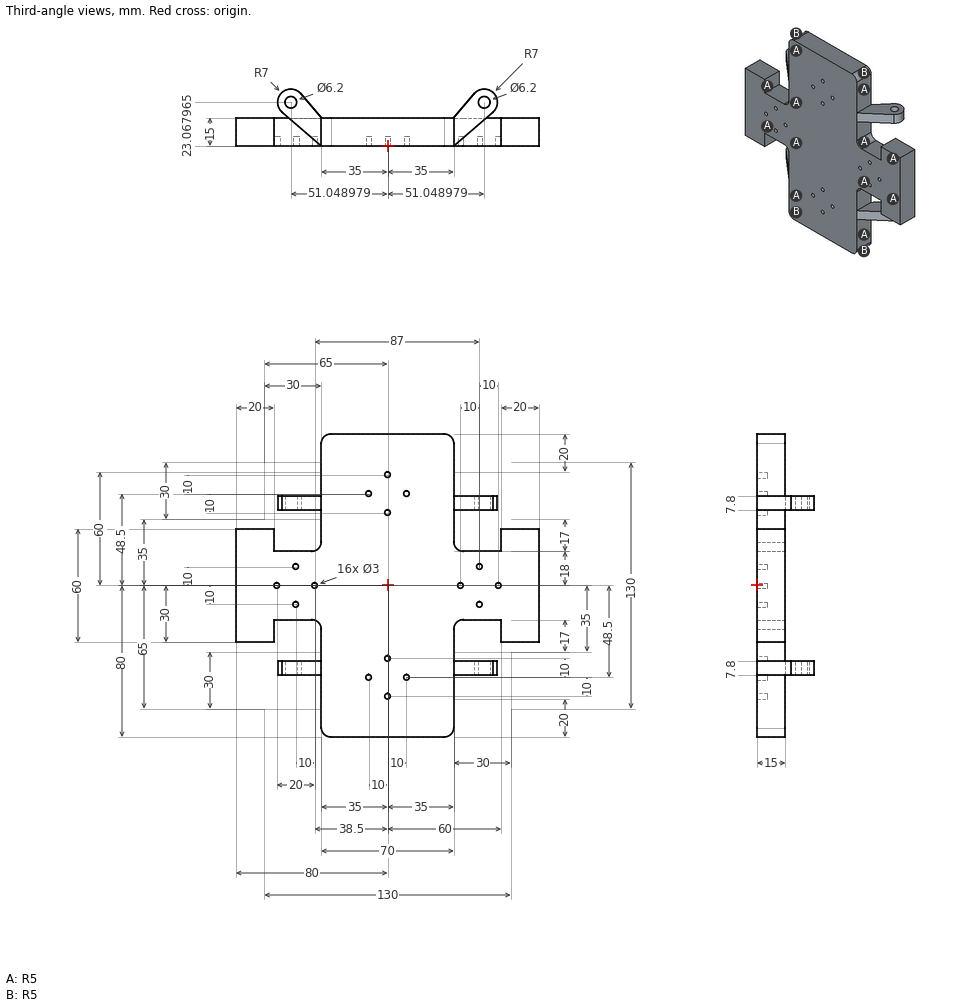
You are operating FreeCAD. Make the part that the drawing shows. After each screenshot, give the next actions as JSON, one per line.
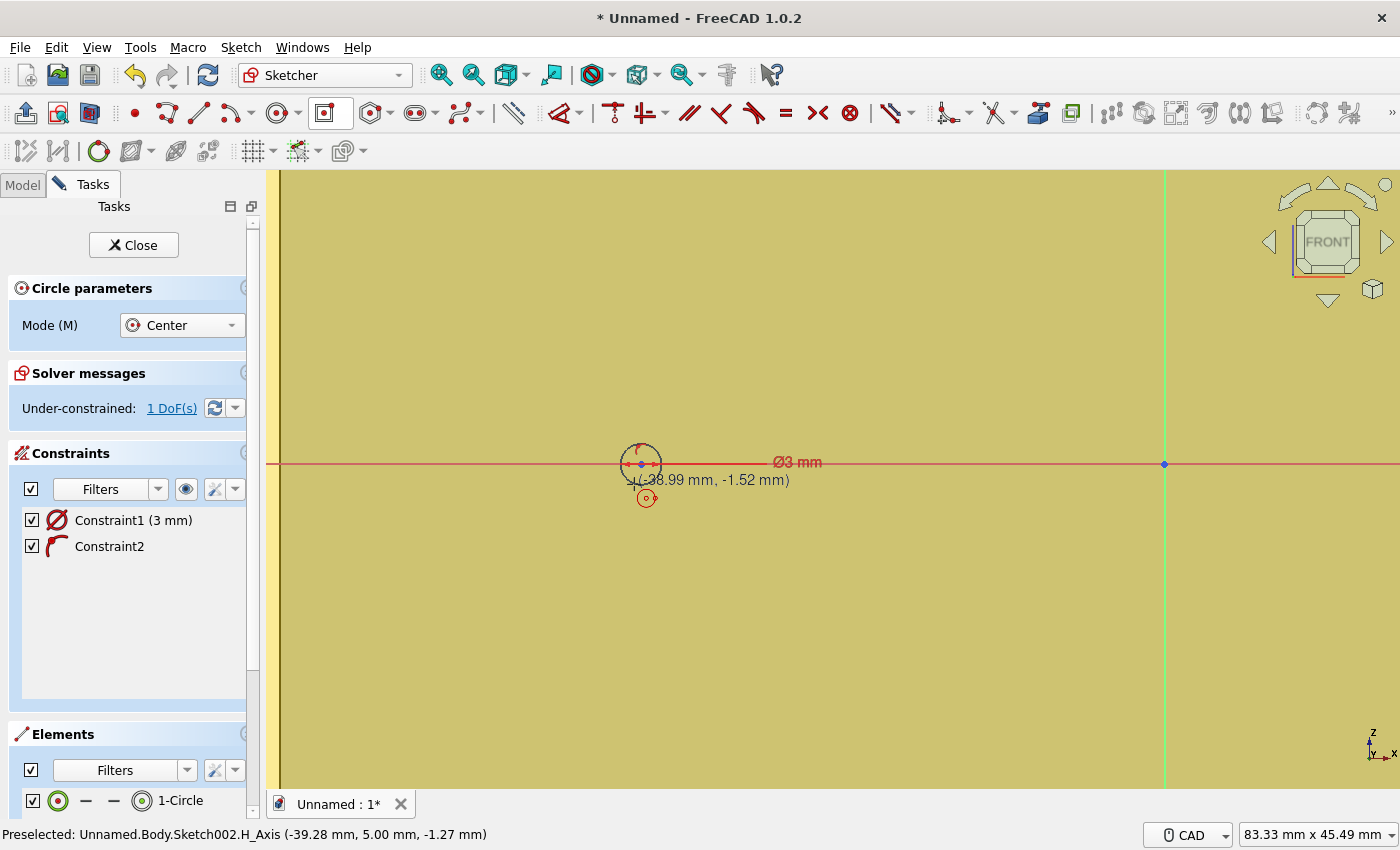
{"action": "scroll", "coordinate": [634, 484], "scroll_direction": "down", "scroll_amount": 7}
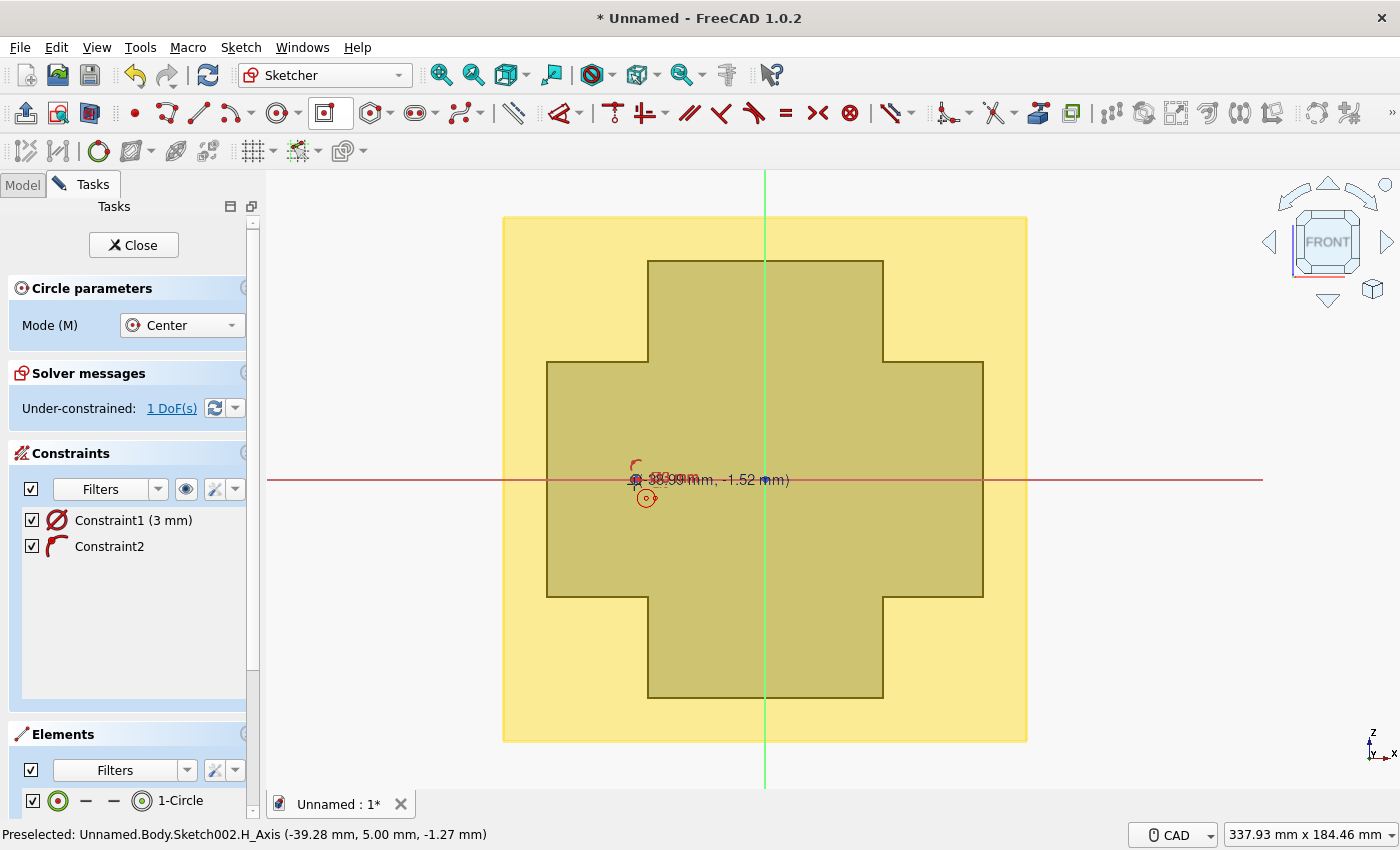
{"action": "left_click", "coordinate": [569, 480]}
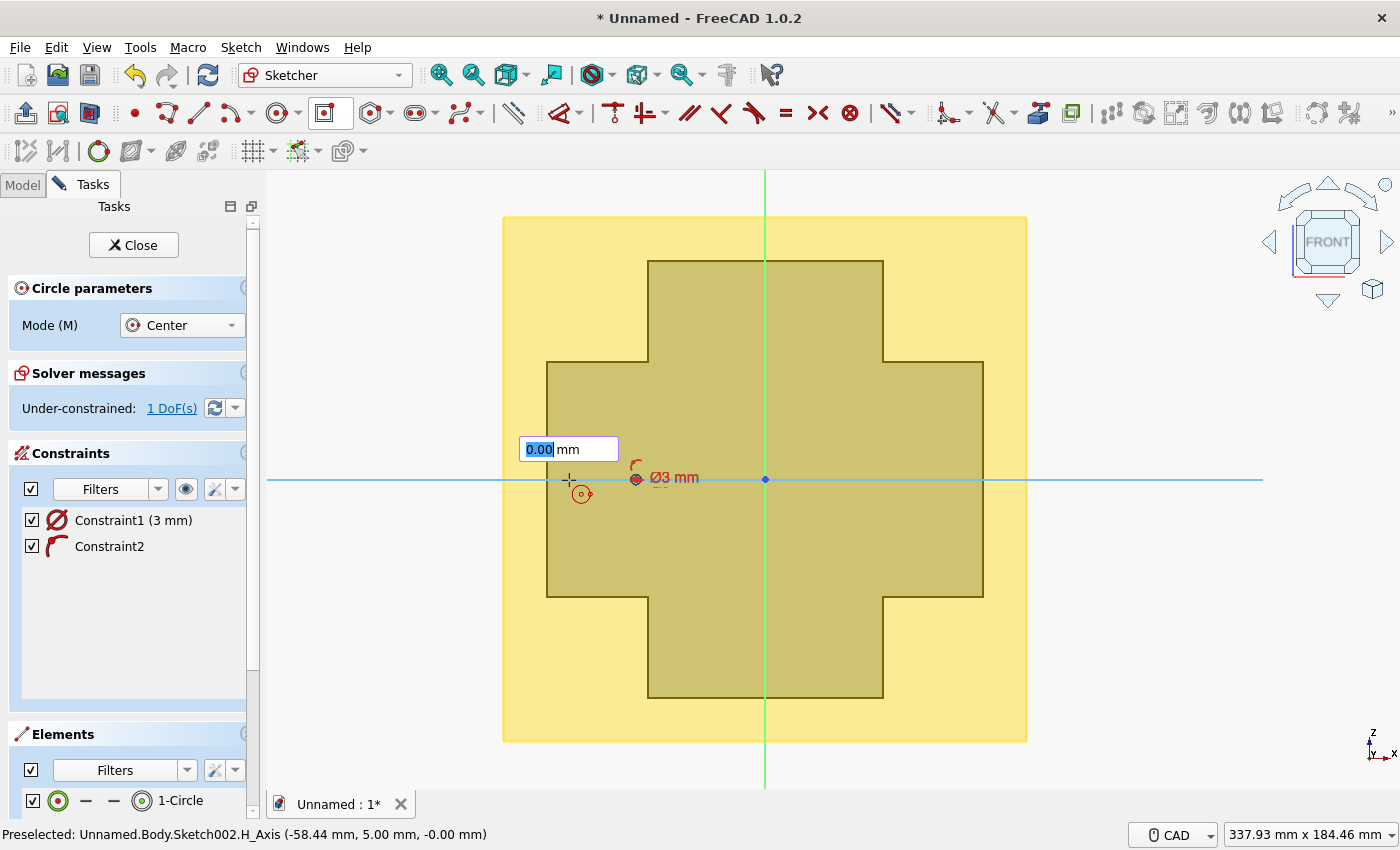
{"action": "scroll", "coordinate": [567, 484], "scroll_direction": "up", "scroll_amount": 7}
{"action": "mouse_move", "coordinate": [566, 484]}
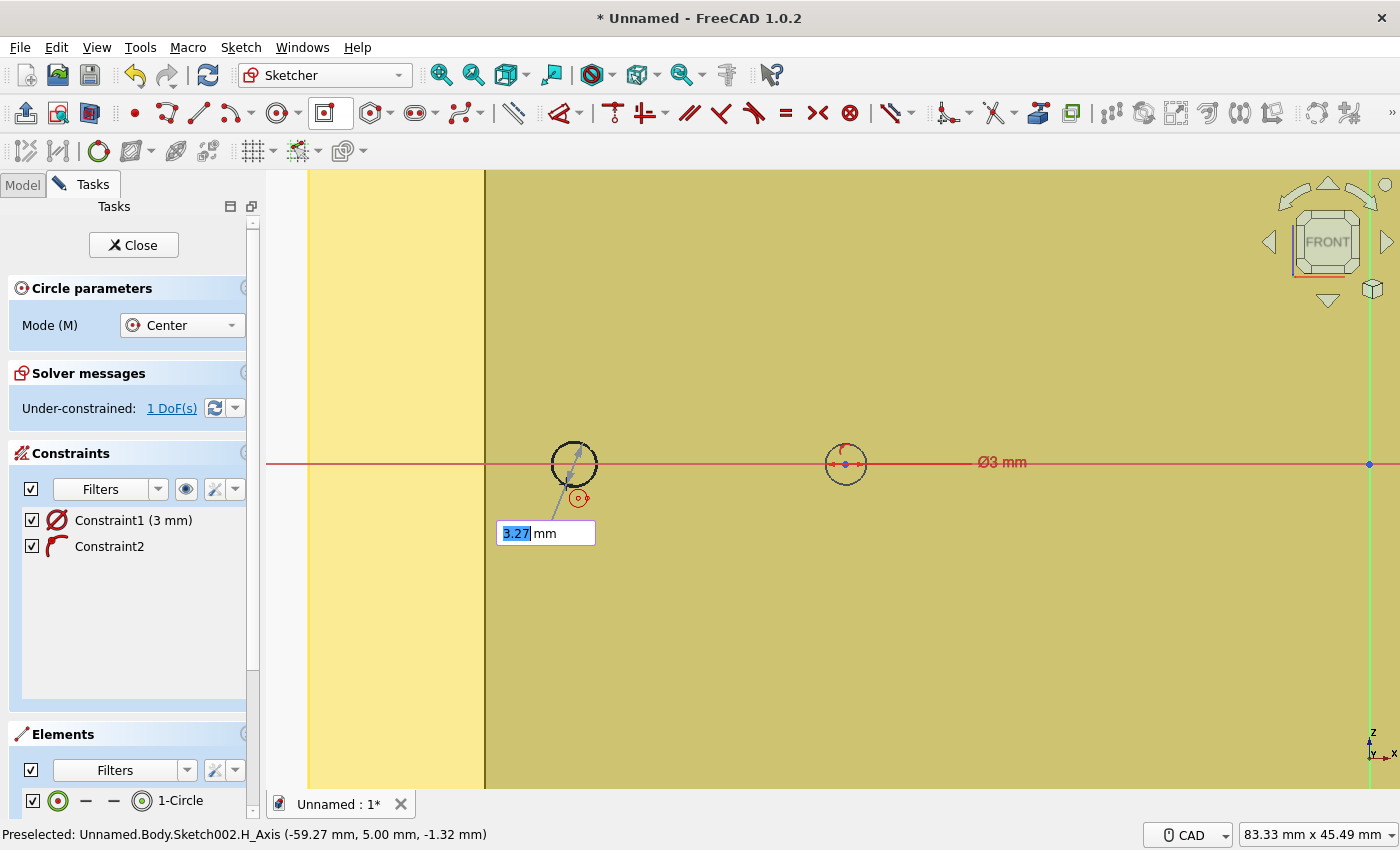
{"action": "type", "text": "3"}
{"action": "key", "text": "Return"}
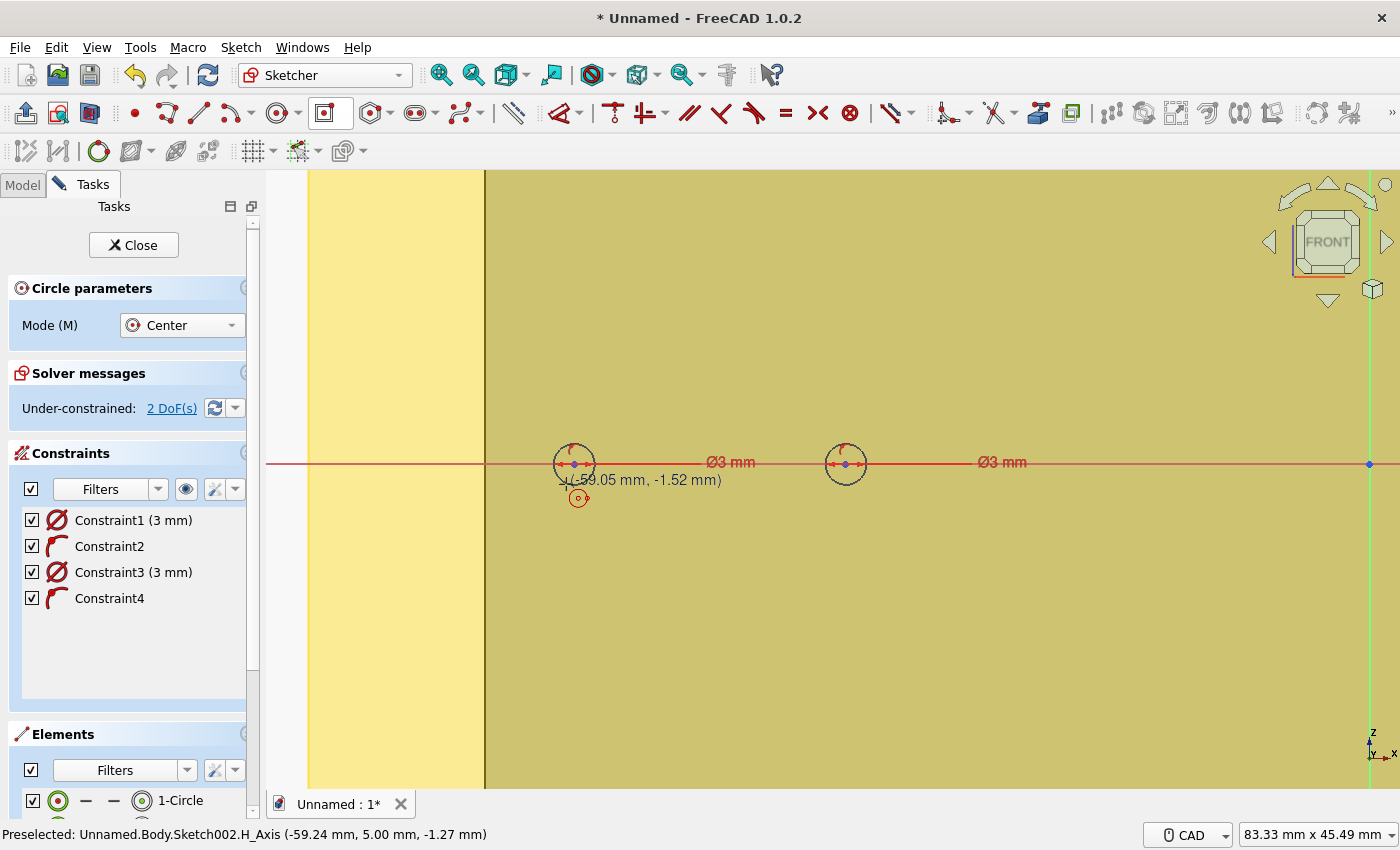
{"action": "scroll", "coordinate": [566, 484], "scroll_direction": "down", "scroll_amount": 7}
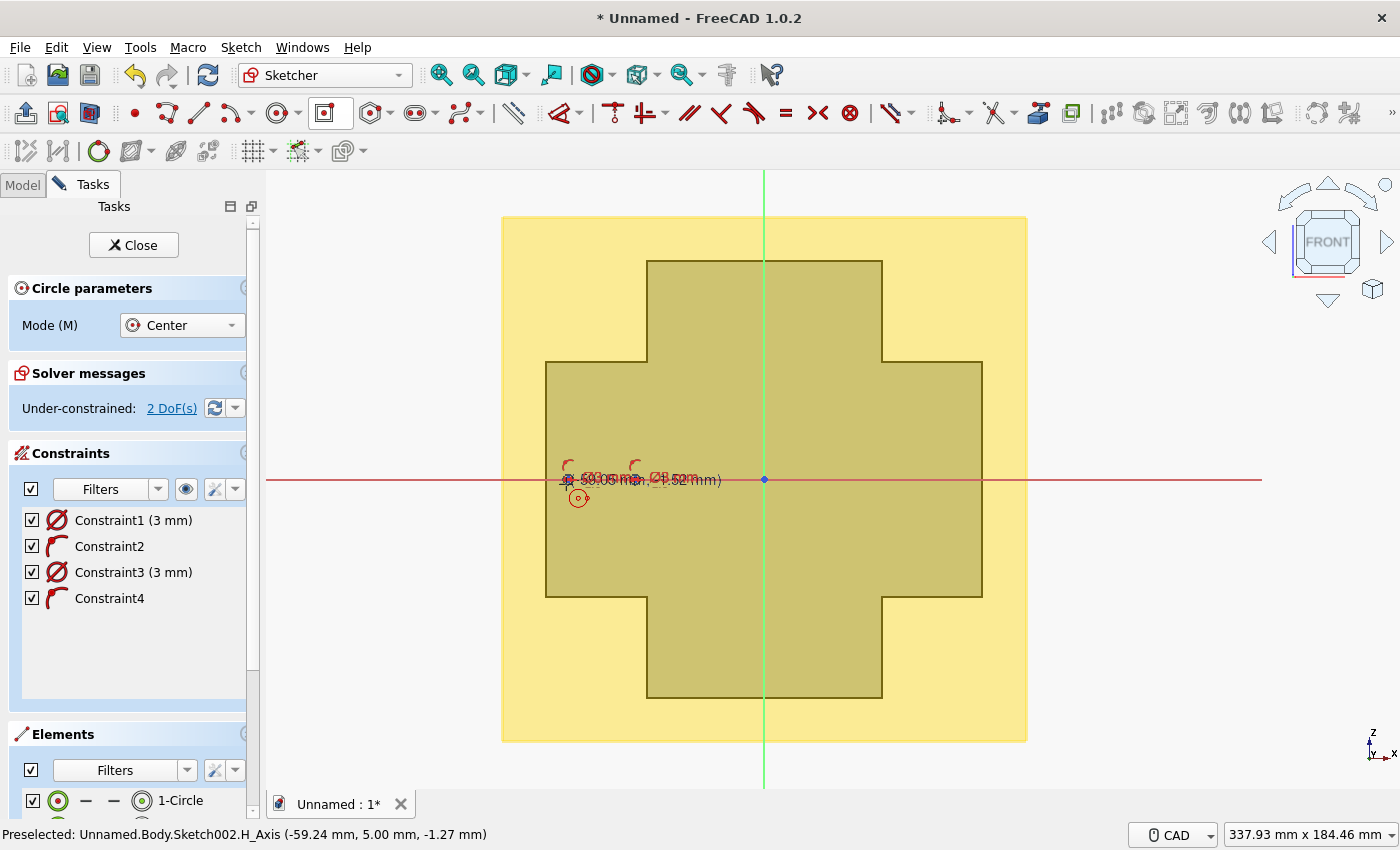
{"action": "left_click", "coordinate": [602, 513]}
{"action": "mouse_move", "coordinate": [605, 510]}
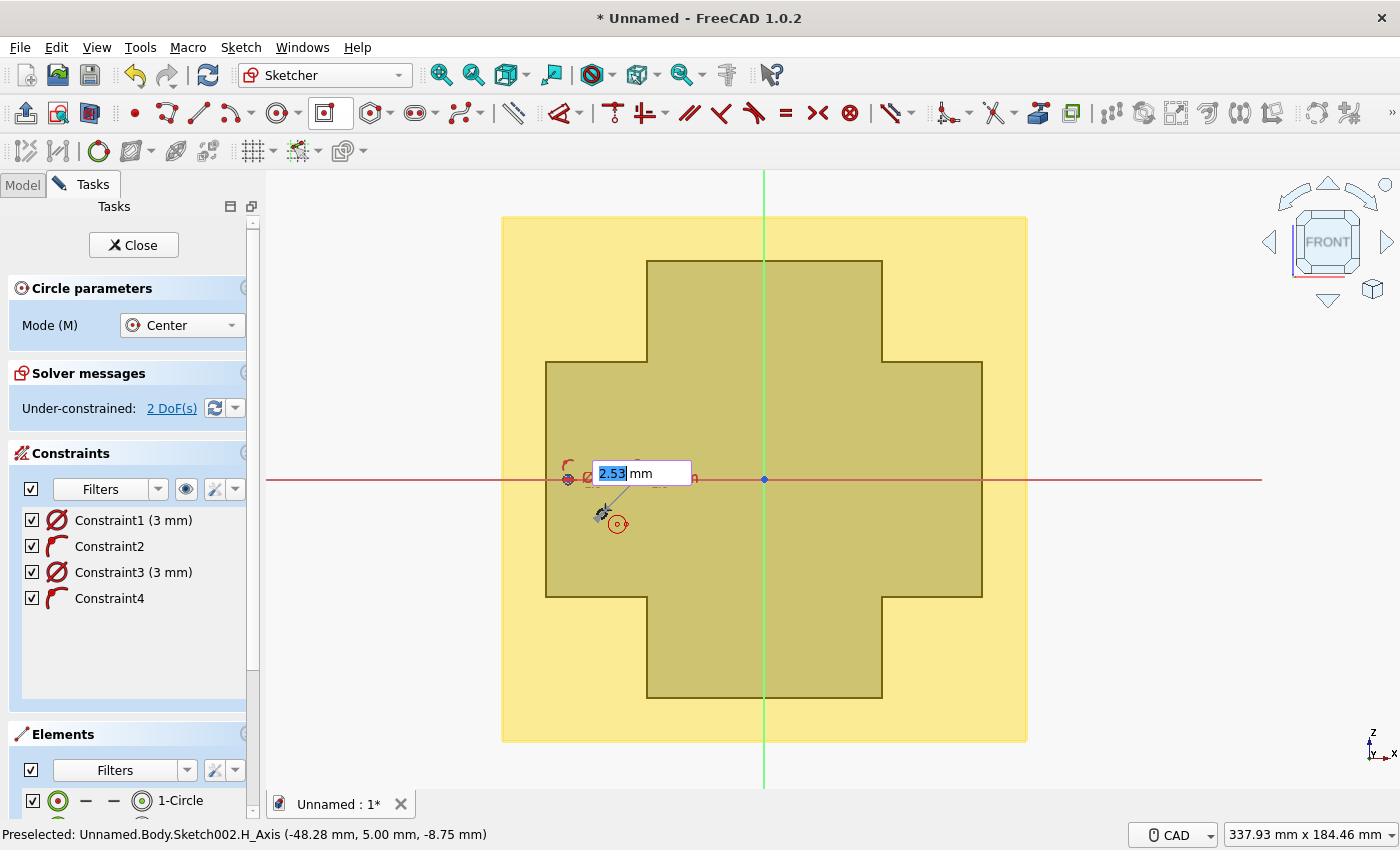
{"action": "type", "text": "3"}
{"action": "key", "text": "Return"}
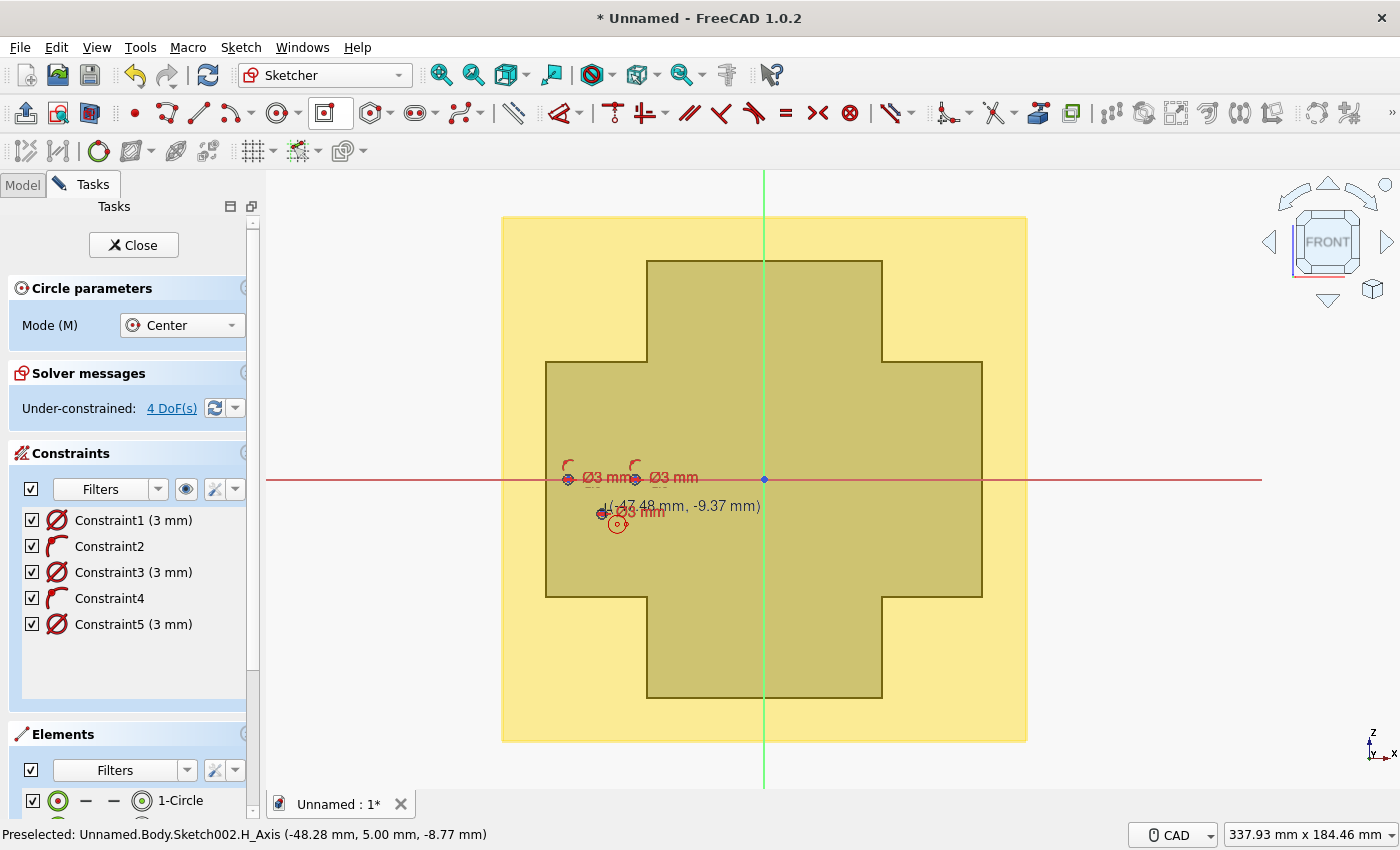
{"action": "scroll", "coordinate": [602, 446], "scroll_direction": "up", "scroll_amount": 8}